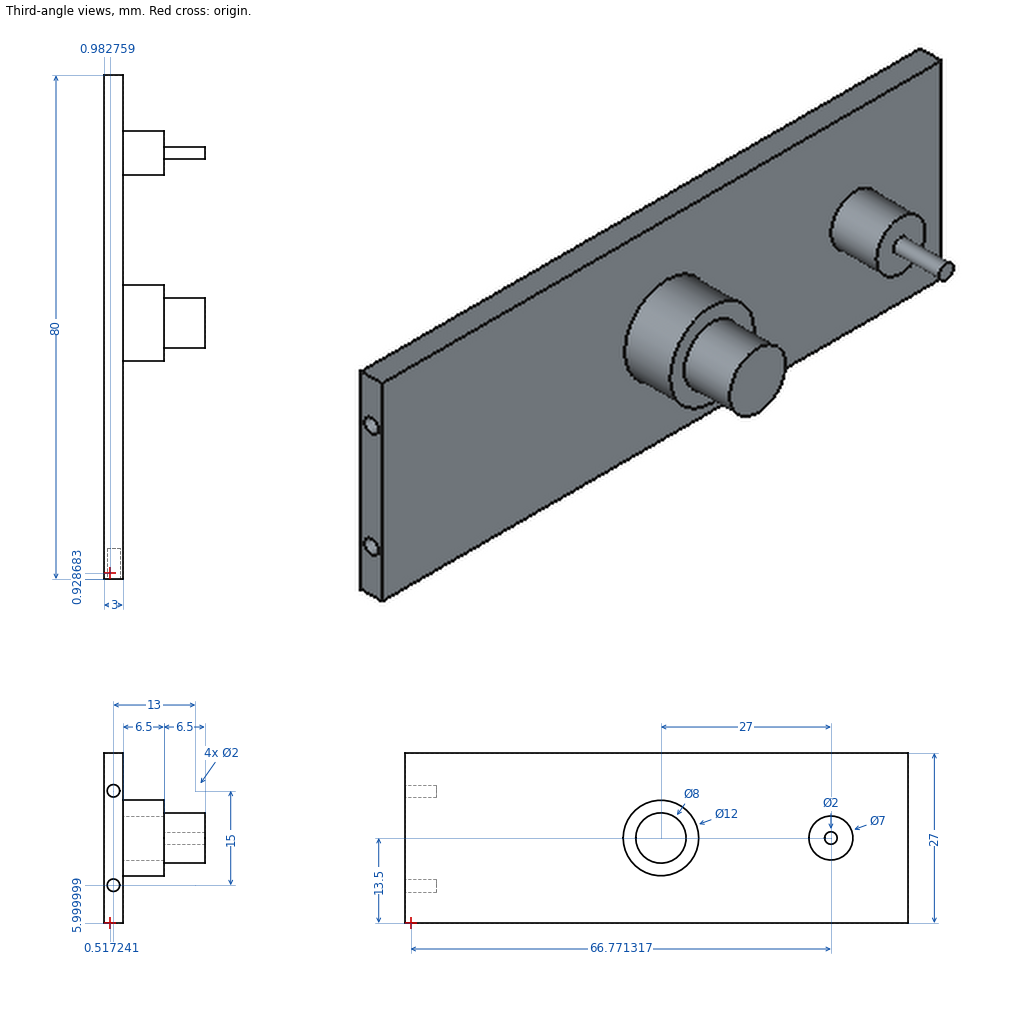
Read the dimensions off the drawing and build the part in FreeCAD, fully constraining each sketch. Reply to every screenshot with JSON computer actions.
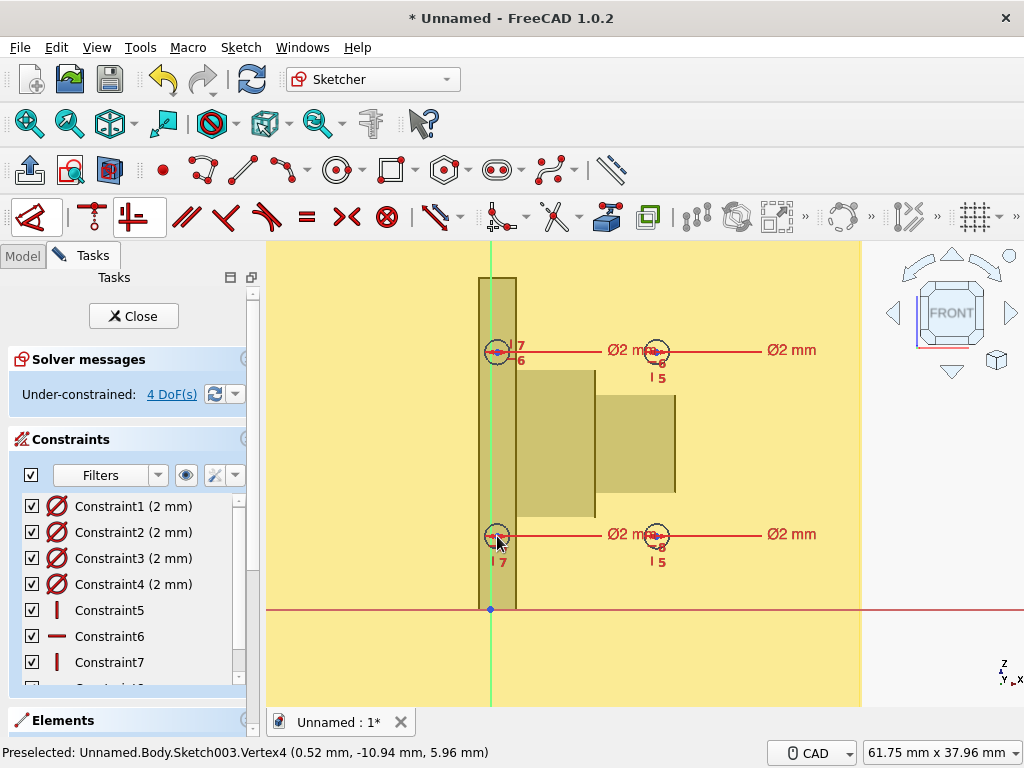
{"action": "left_click", "coordinate": [657, 352]}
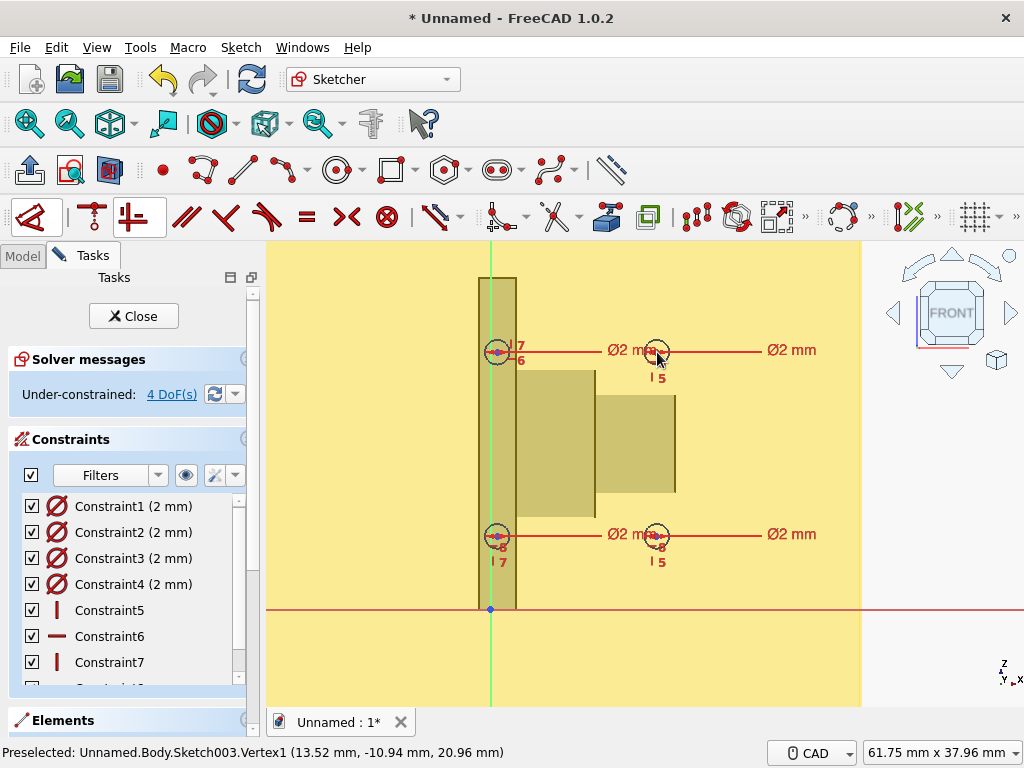
{"action": "left_click", "coordinate": [657, 536]}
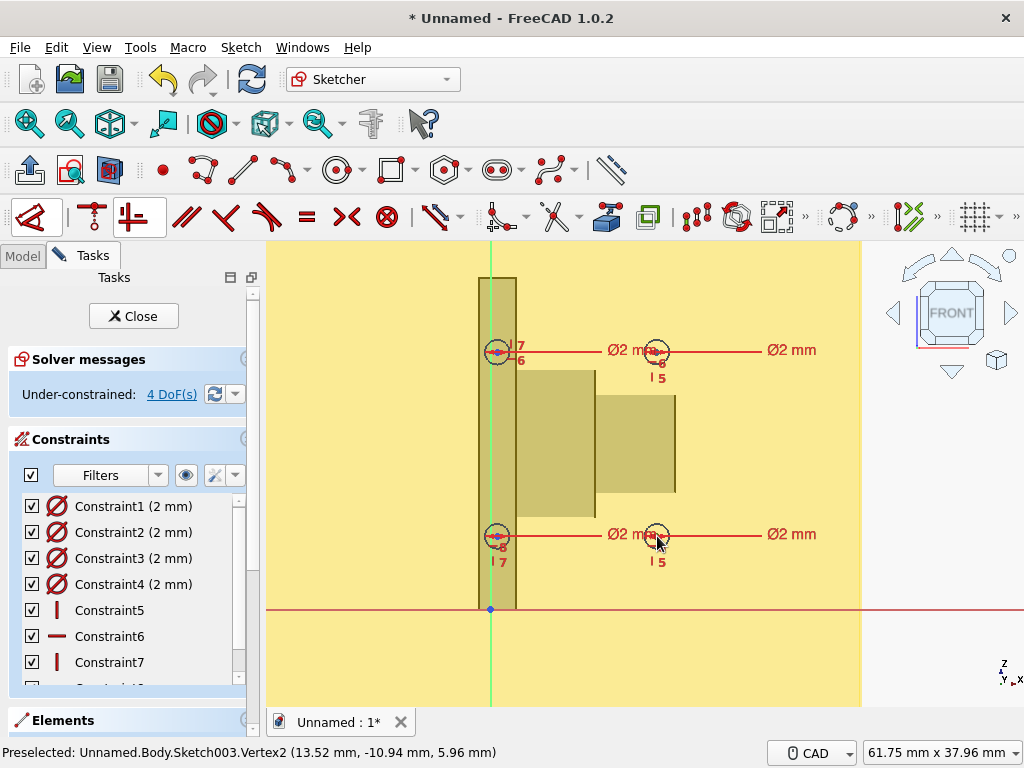
{"action": "key", "text": "i"}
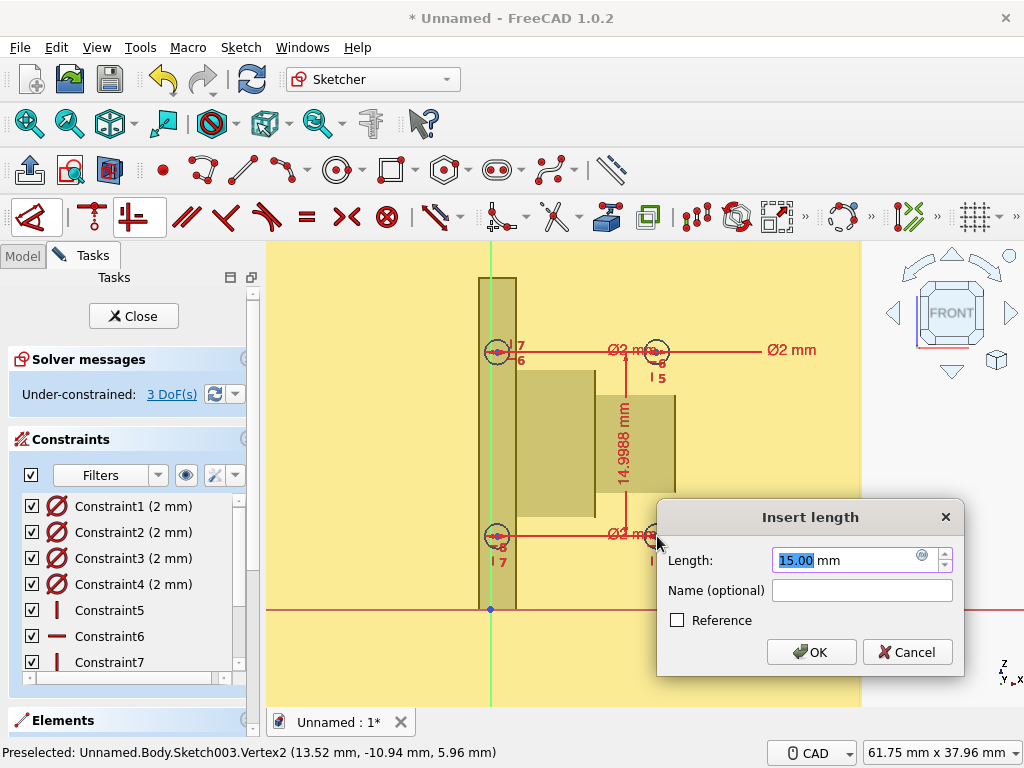
{"action": "type", "text": "15"}
{"action": "key", "text": "Return"}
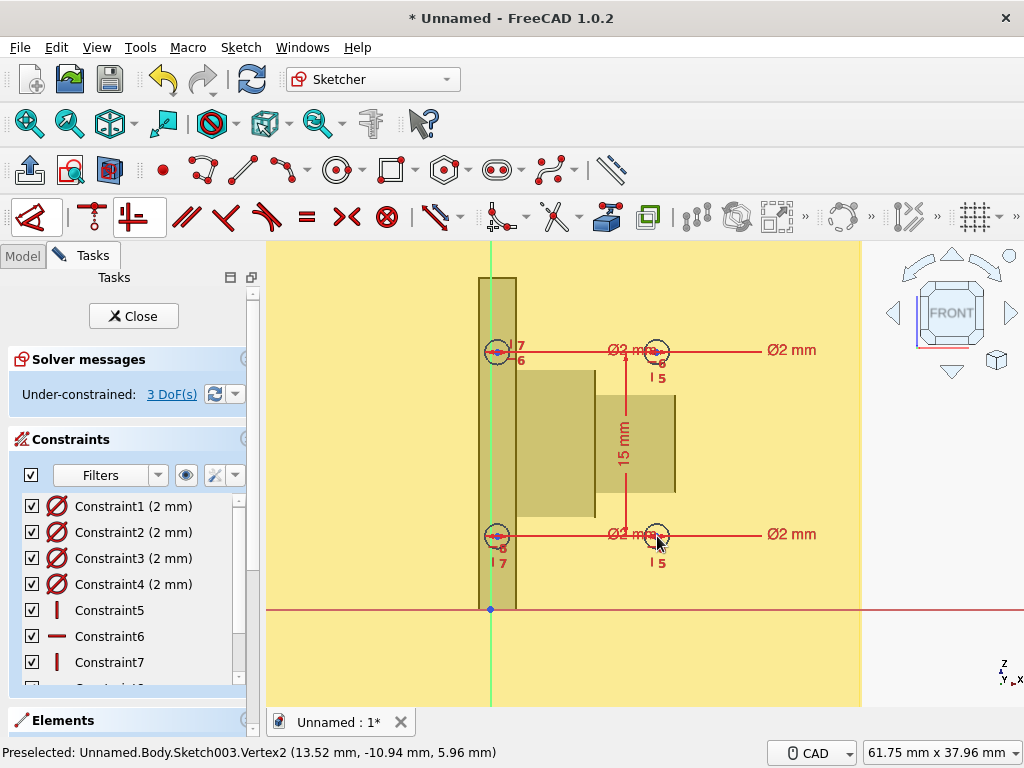
{"action": "left_click", "coordinate": [657, 352]}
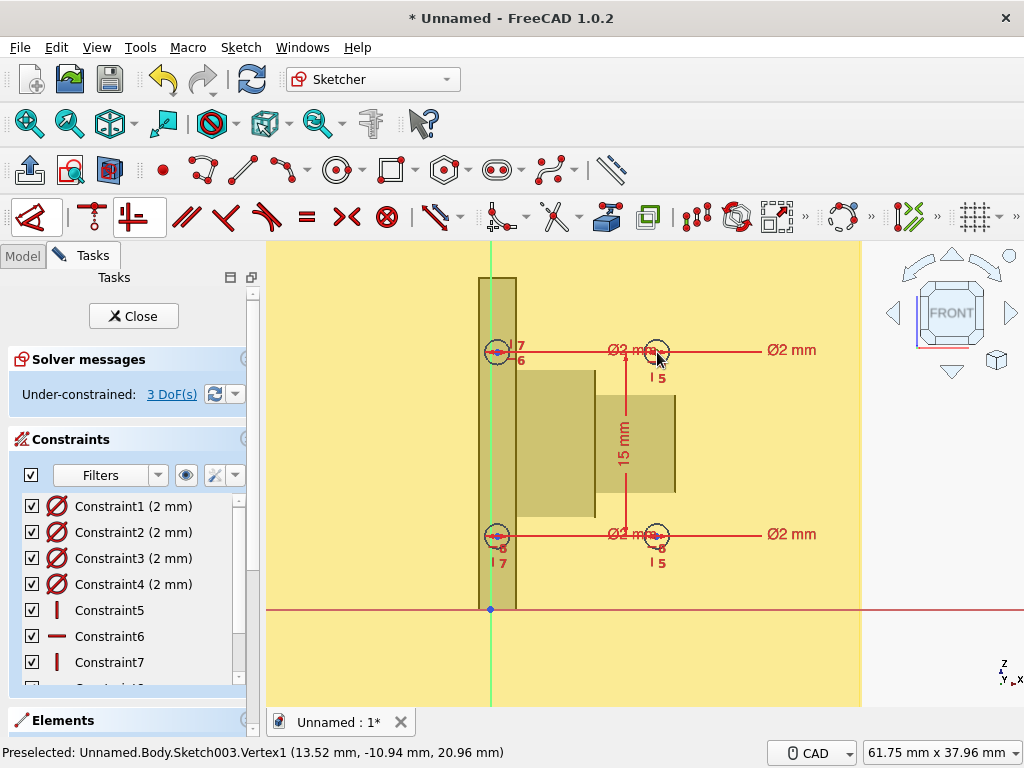
{"action": "left_click", "coordinate": [497, 352]}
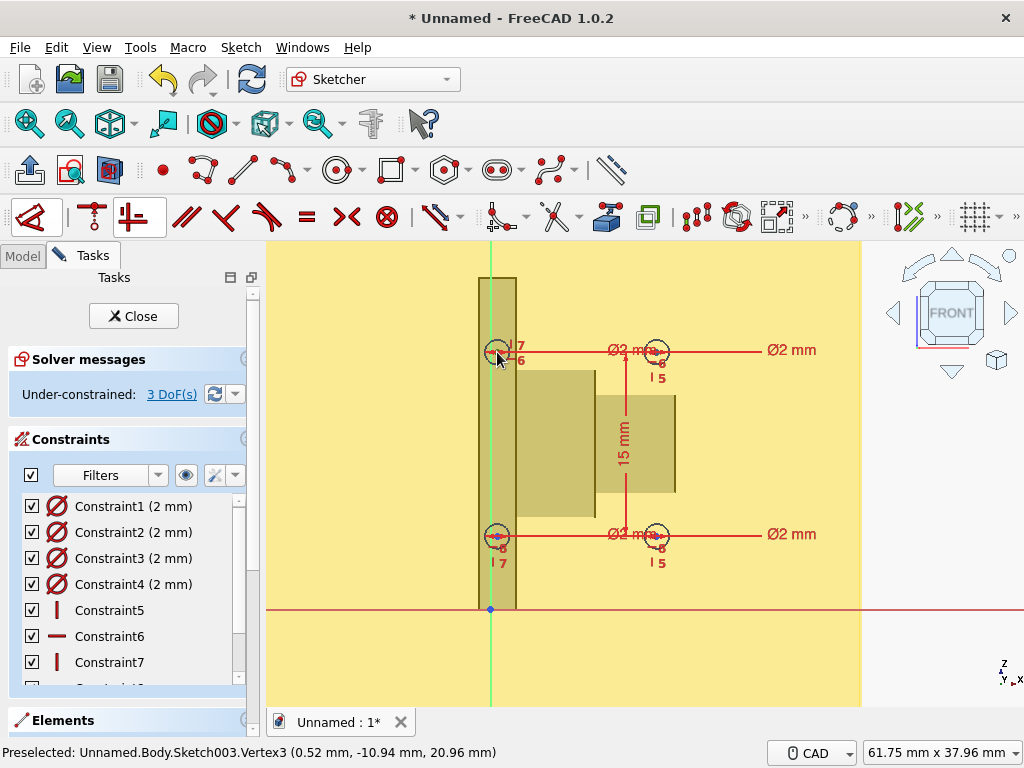
{"action": "key", "text": "l"}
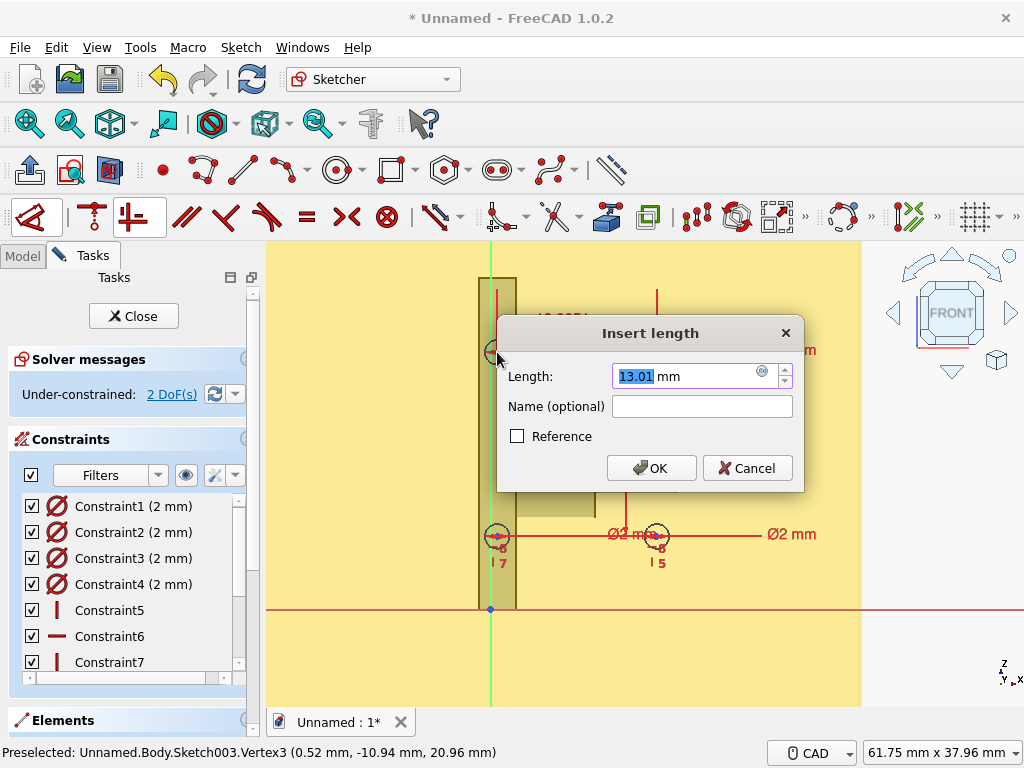
{"action": "type", "text": "13"}
{"action": "key", "text": "Return"}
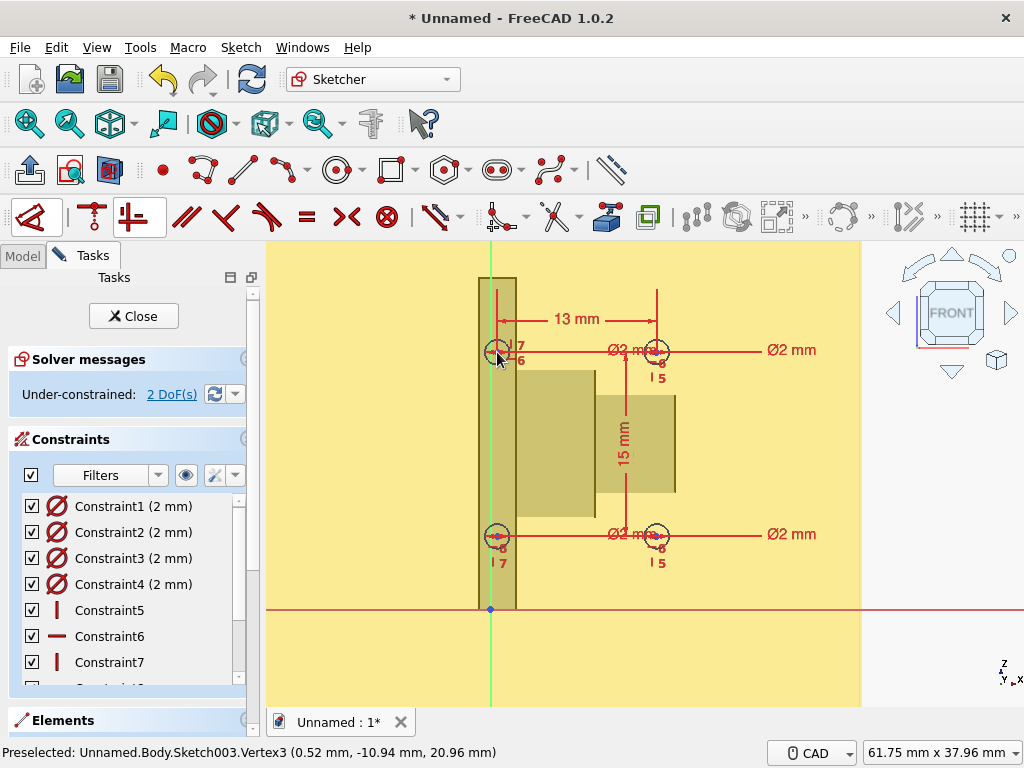
{"action": "left_click", "coordinate": [657, 536]}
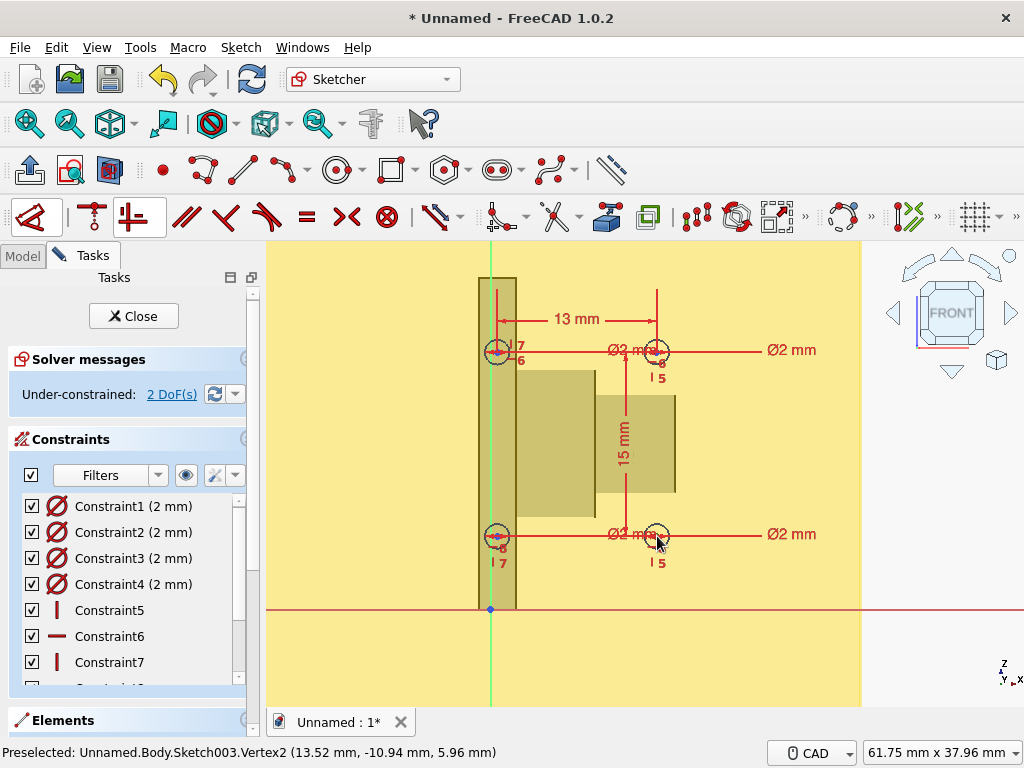
{"action": "key", "text": "i"}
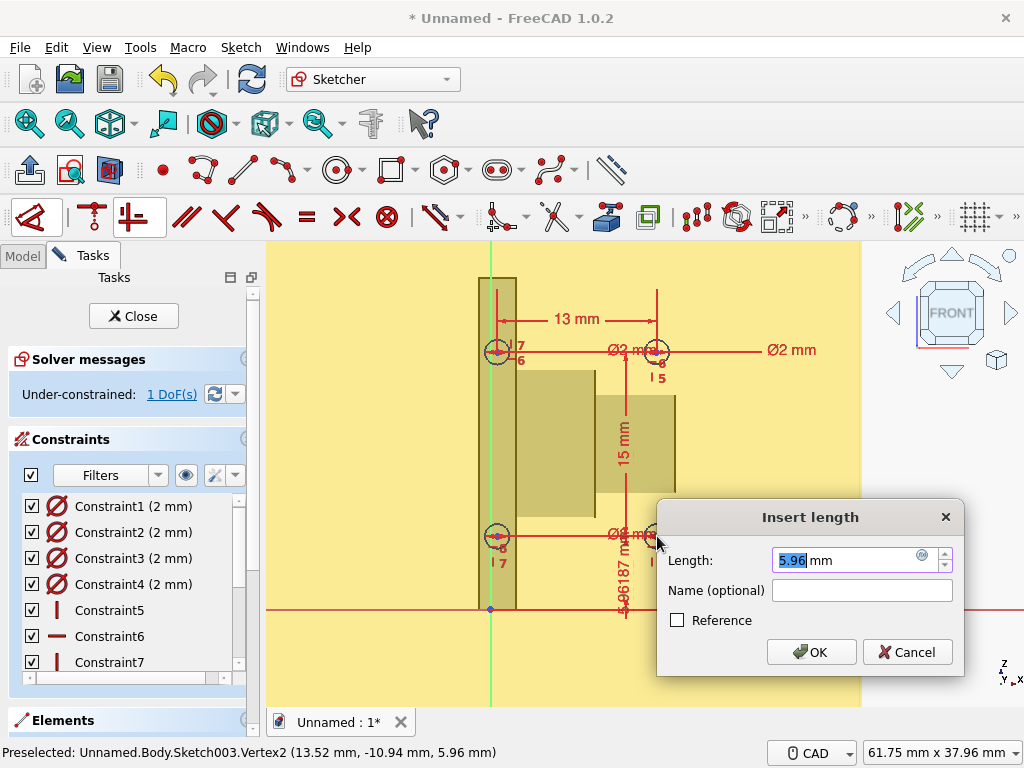
{"action": "type", "text": "5.999999"}
{"action": "key", "text": "Return"}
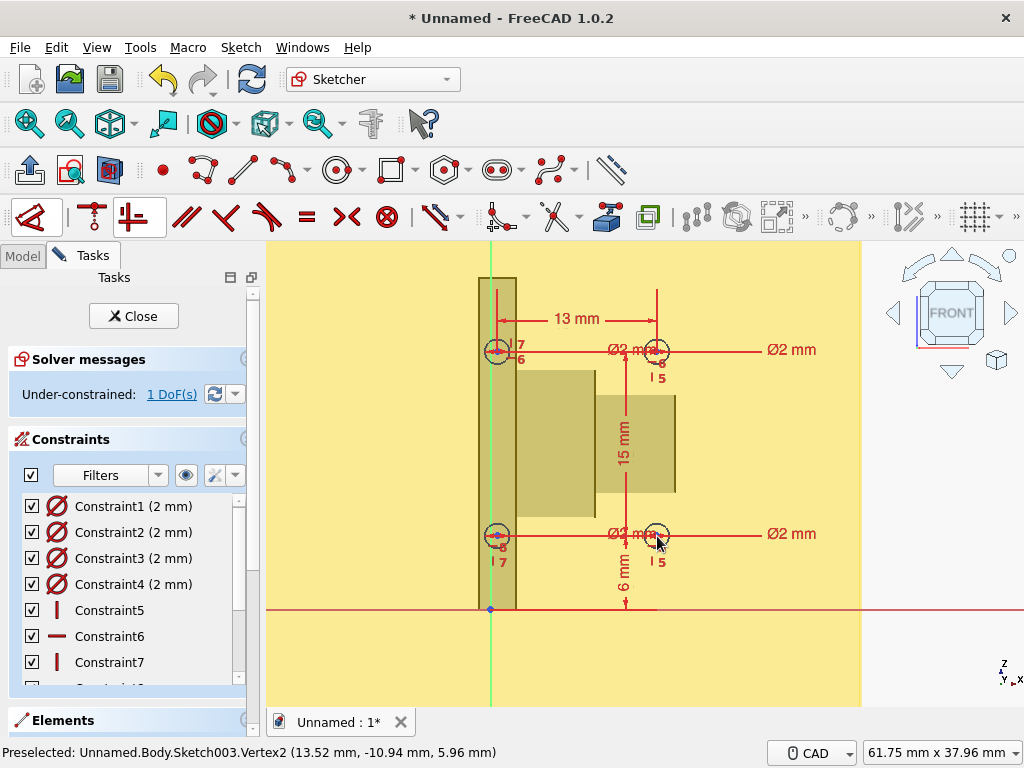
{"action": "scroll", "coordinate": [497, 352], "scroll_direction": "up", "scroll_amount": 10}